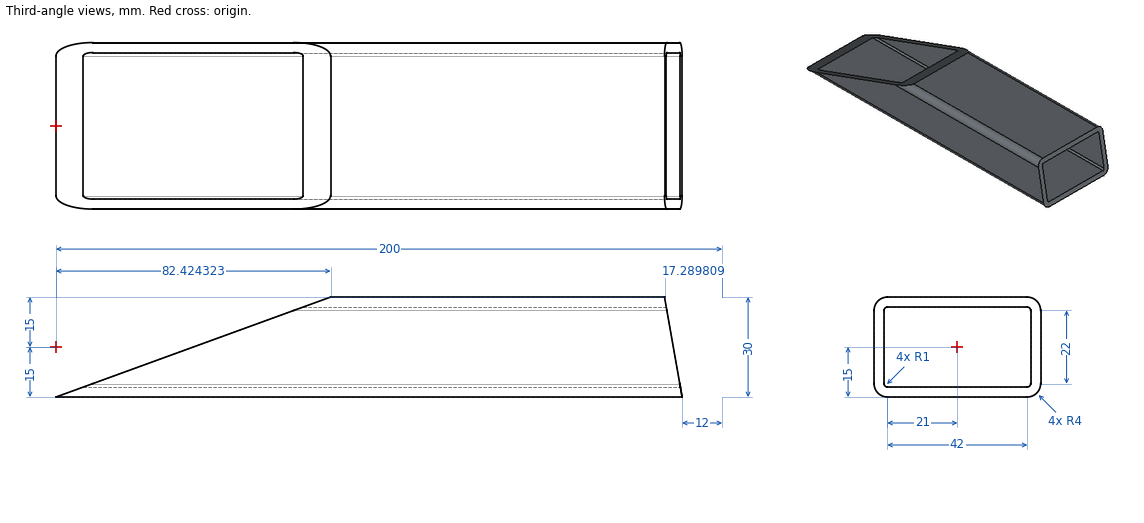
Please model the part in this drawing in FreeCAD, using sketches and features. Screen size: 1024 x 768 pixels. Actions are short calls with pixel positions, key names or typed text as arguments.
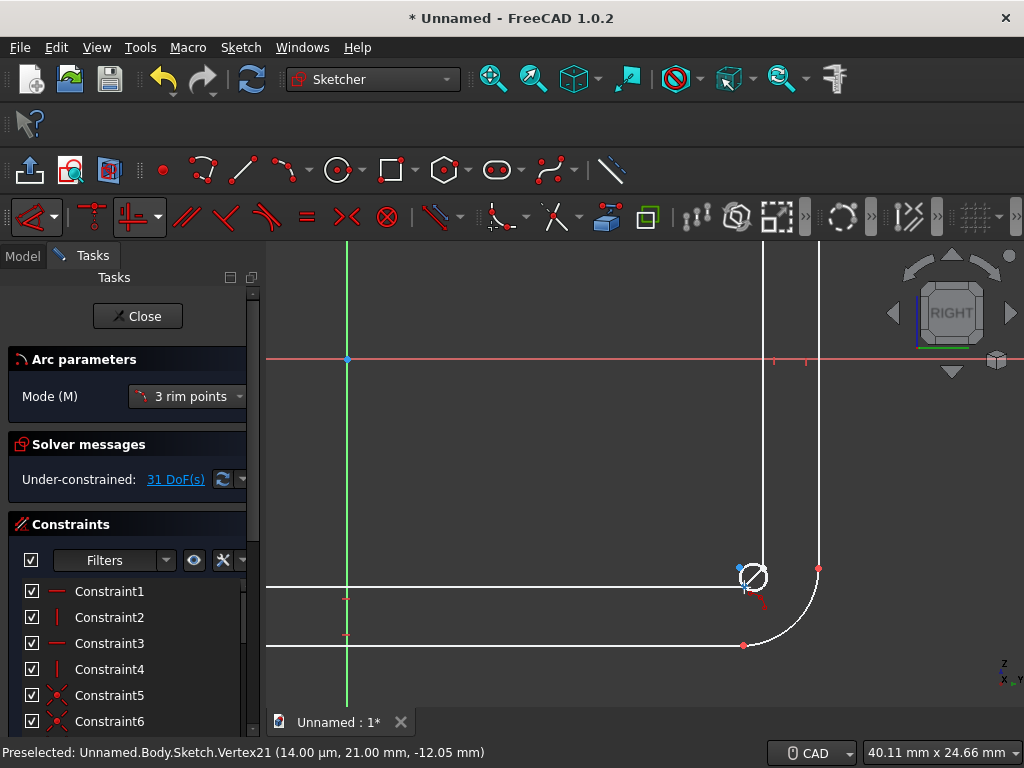
scroll(757, 580, up, 6)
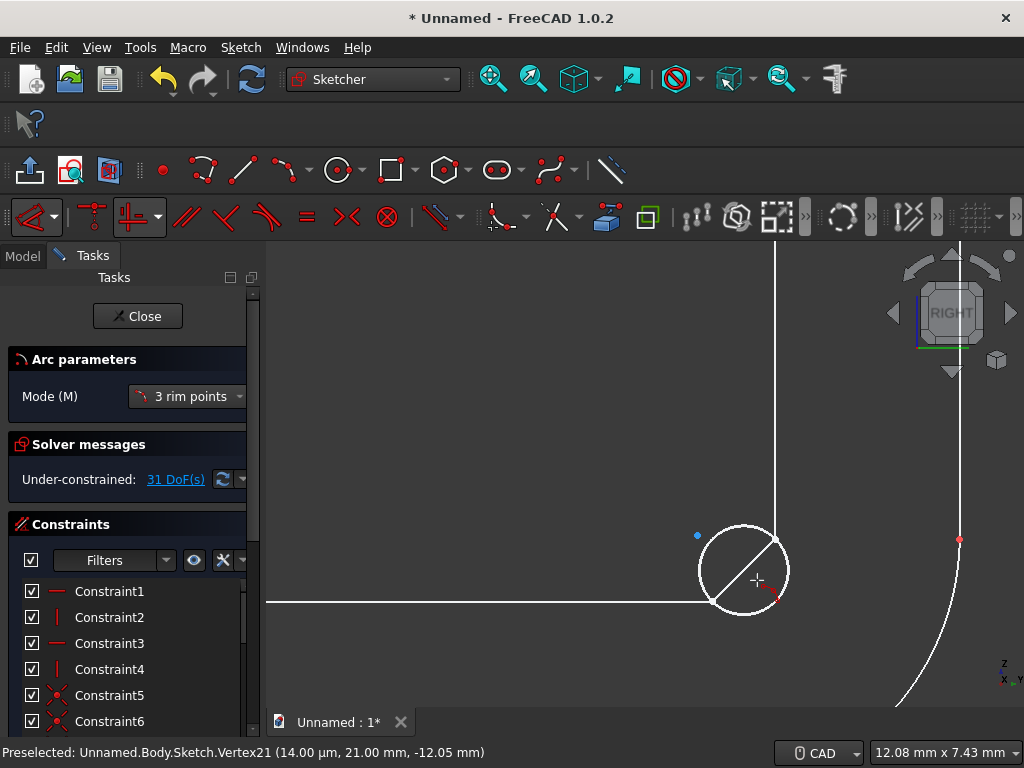
click(756, 580)
key(Escape)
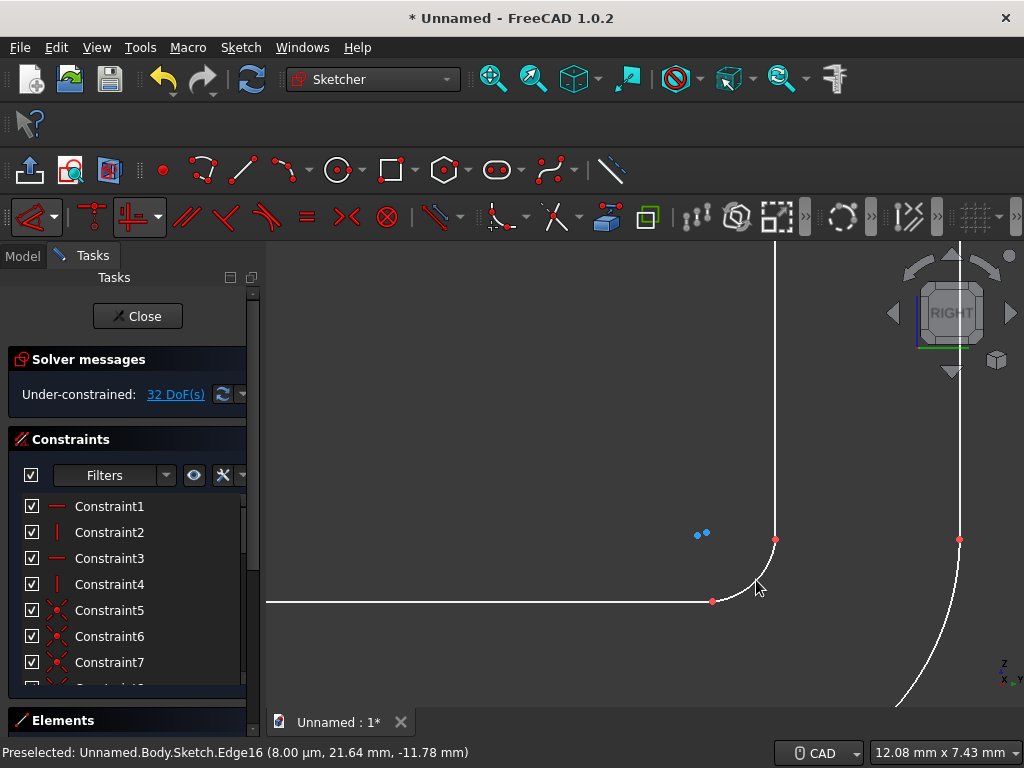
scroll(761, 572, down, 10)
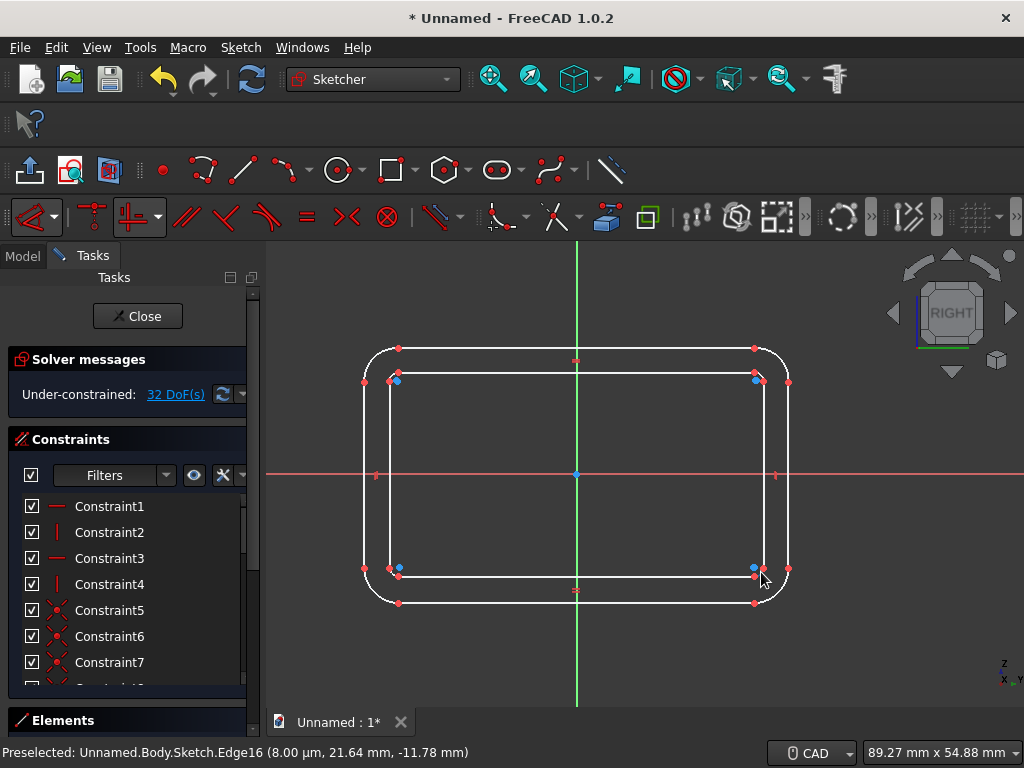
click(505, 603)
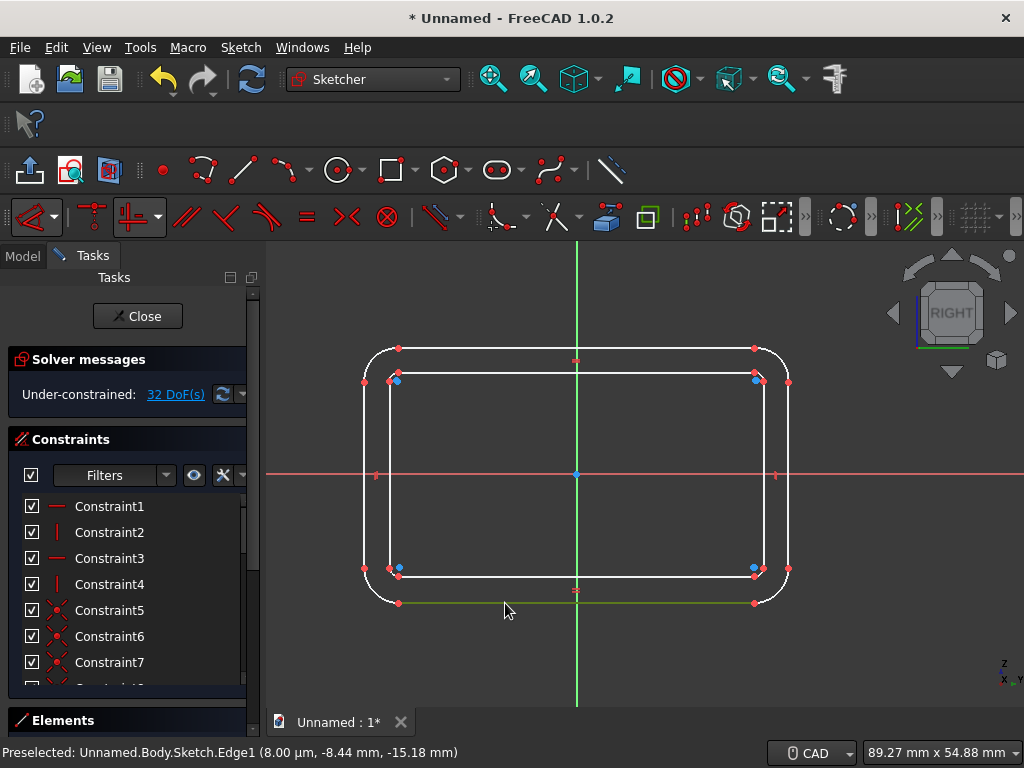
click(770, 599)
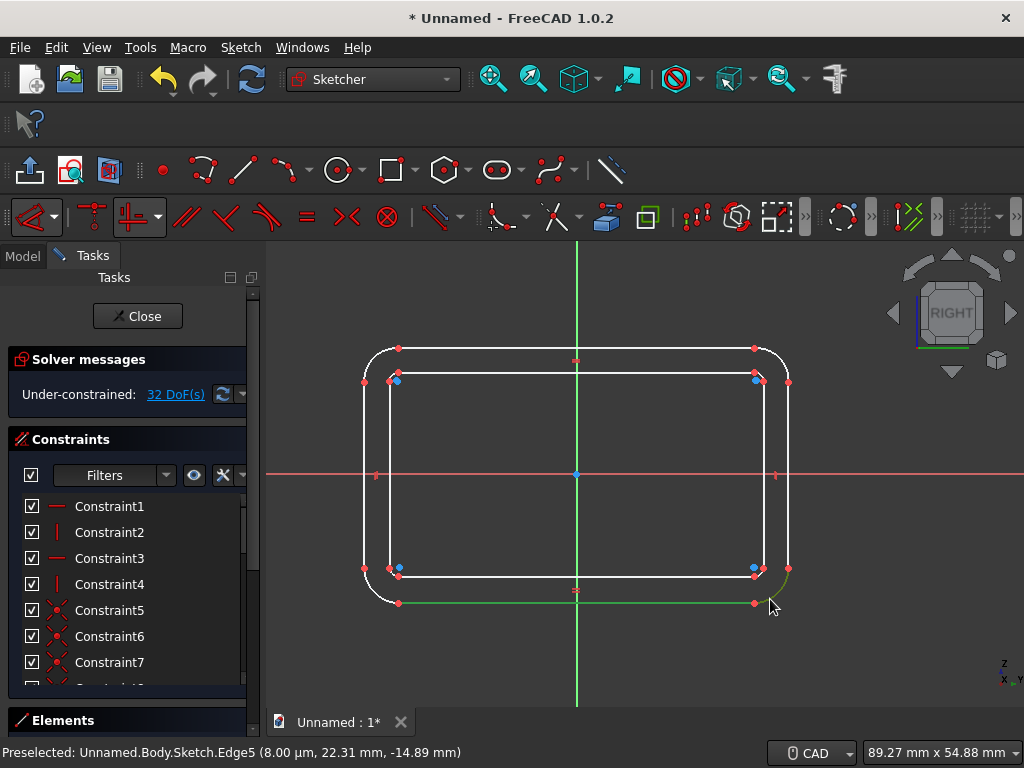
click(268, 218)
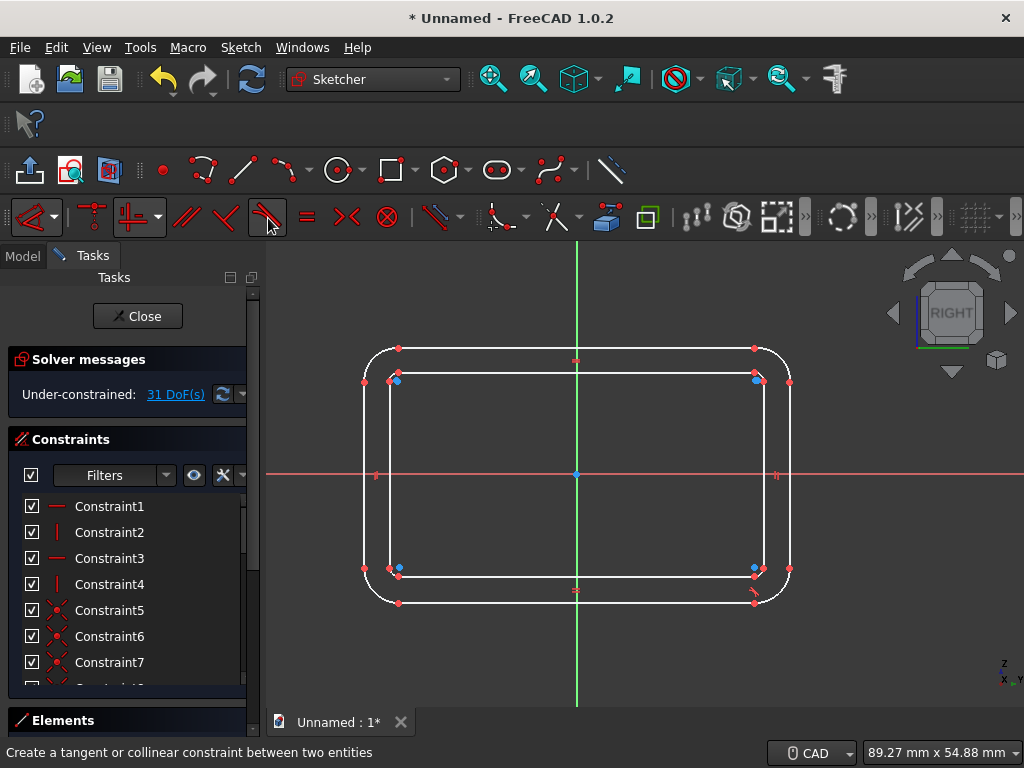
click(505, 603)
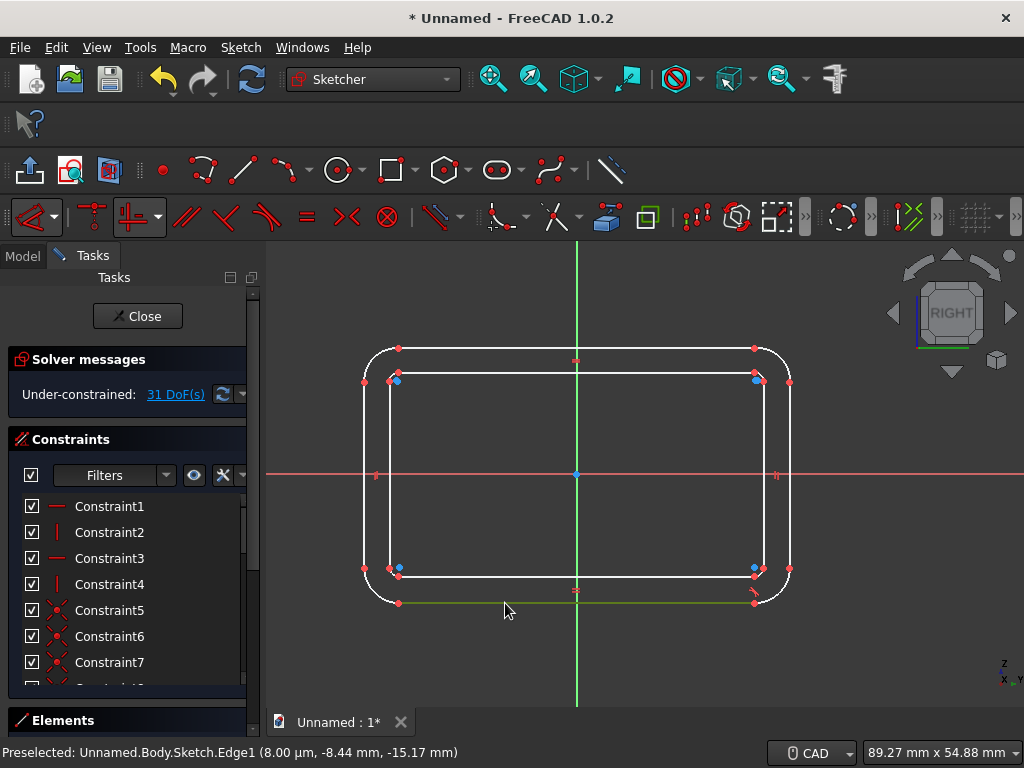
click(368, 584)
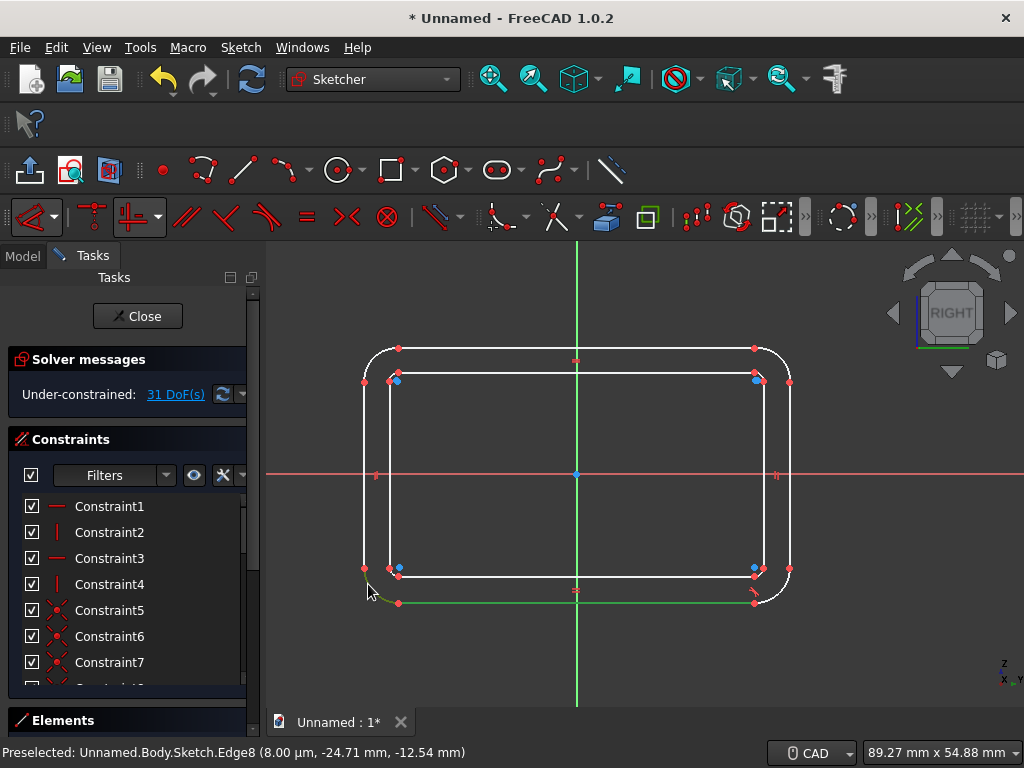
click(268, 218)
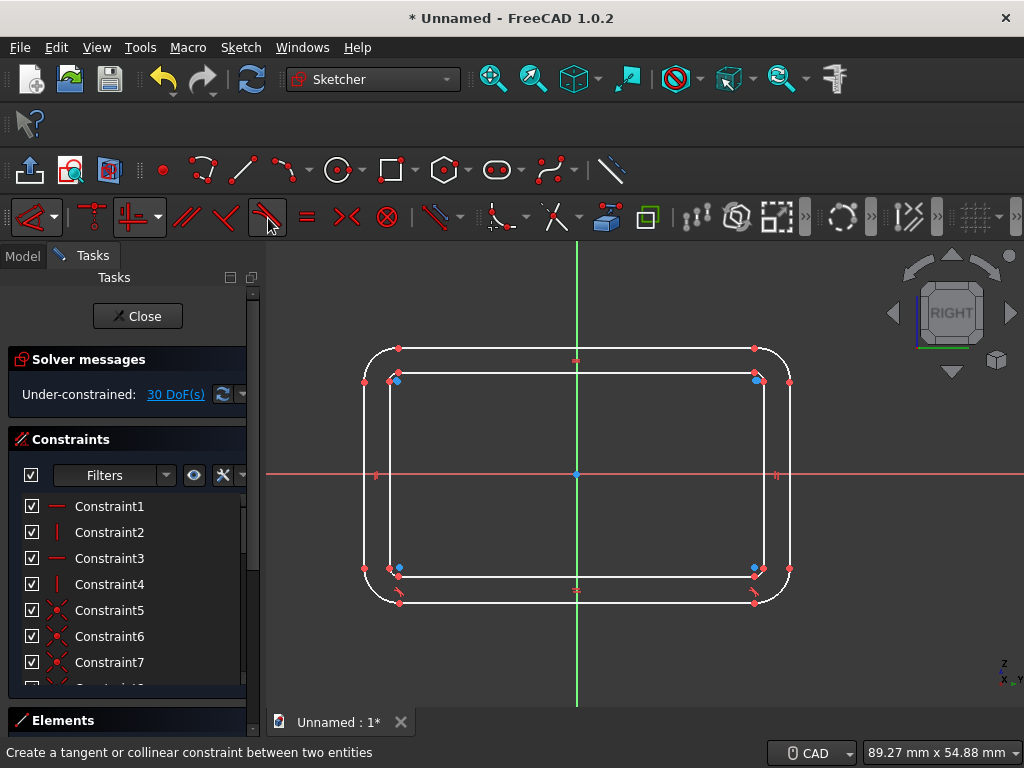
click(790, 512)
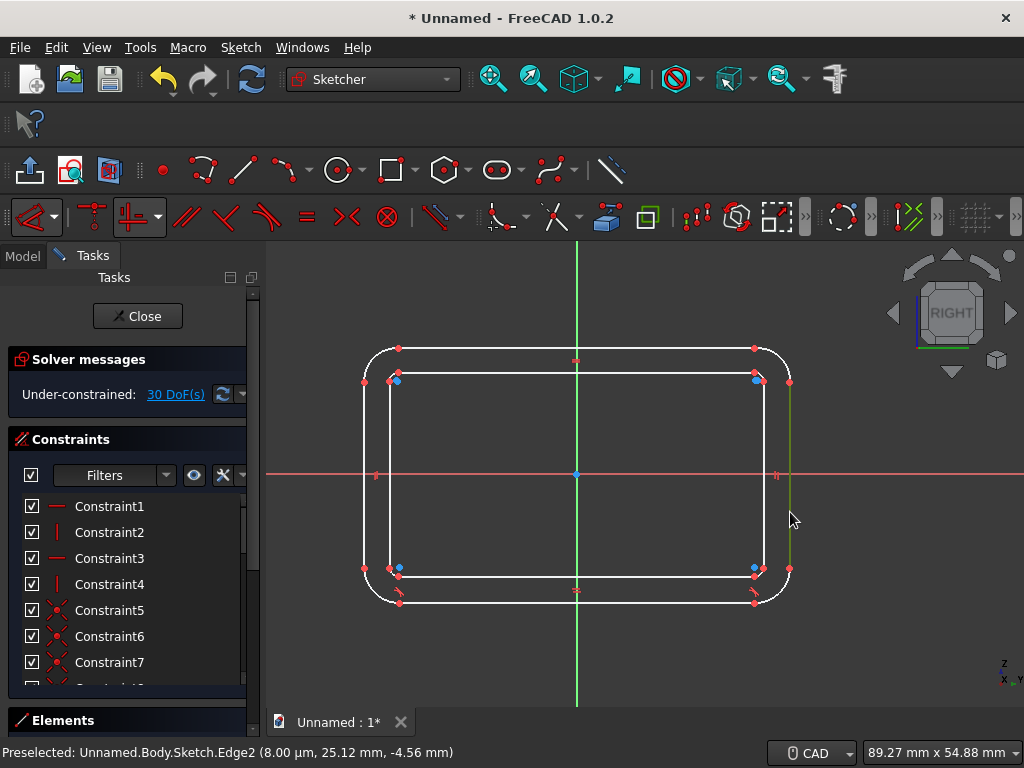
click(770, 599)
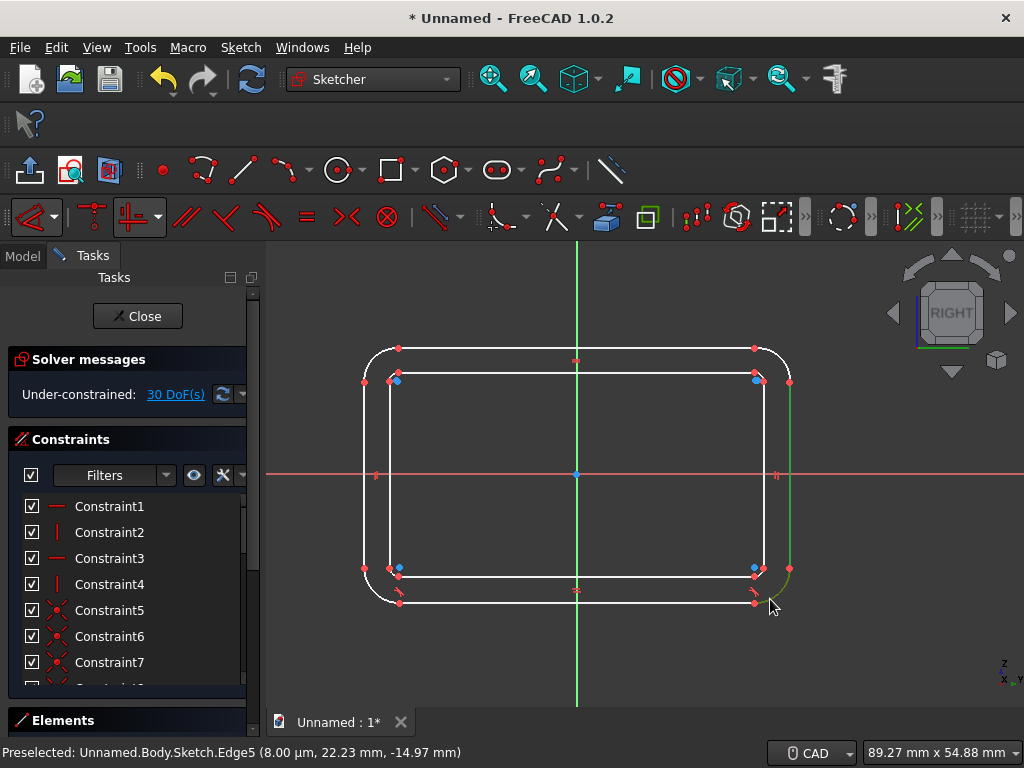
click(268, 218)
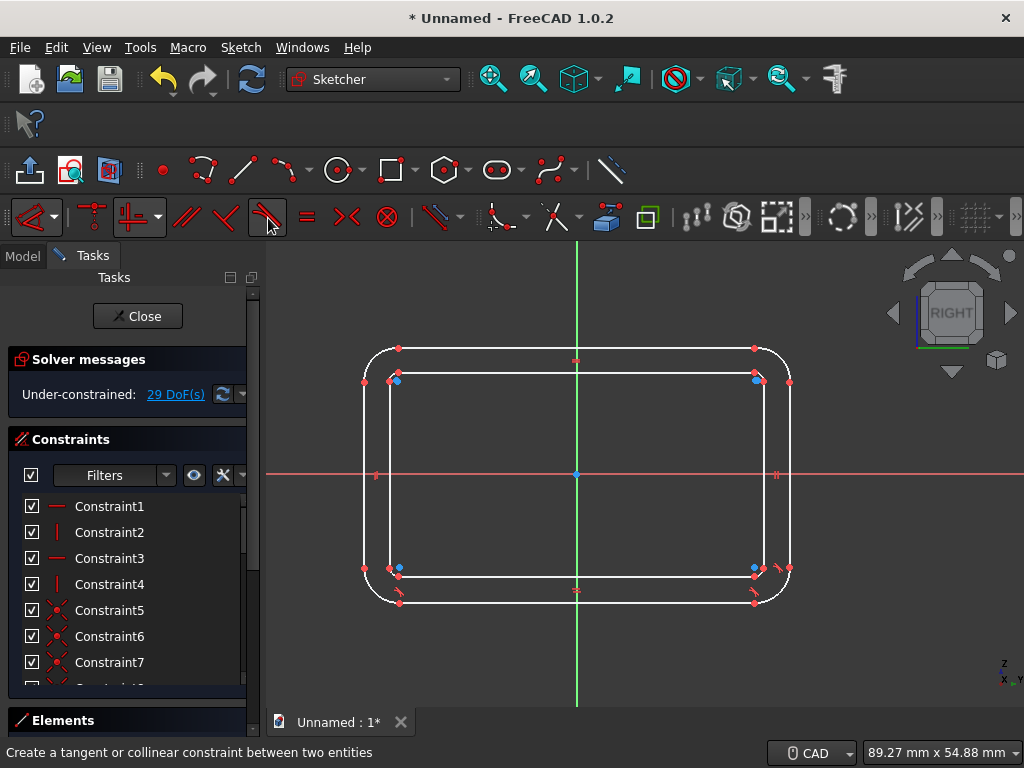
click(790, 512)